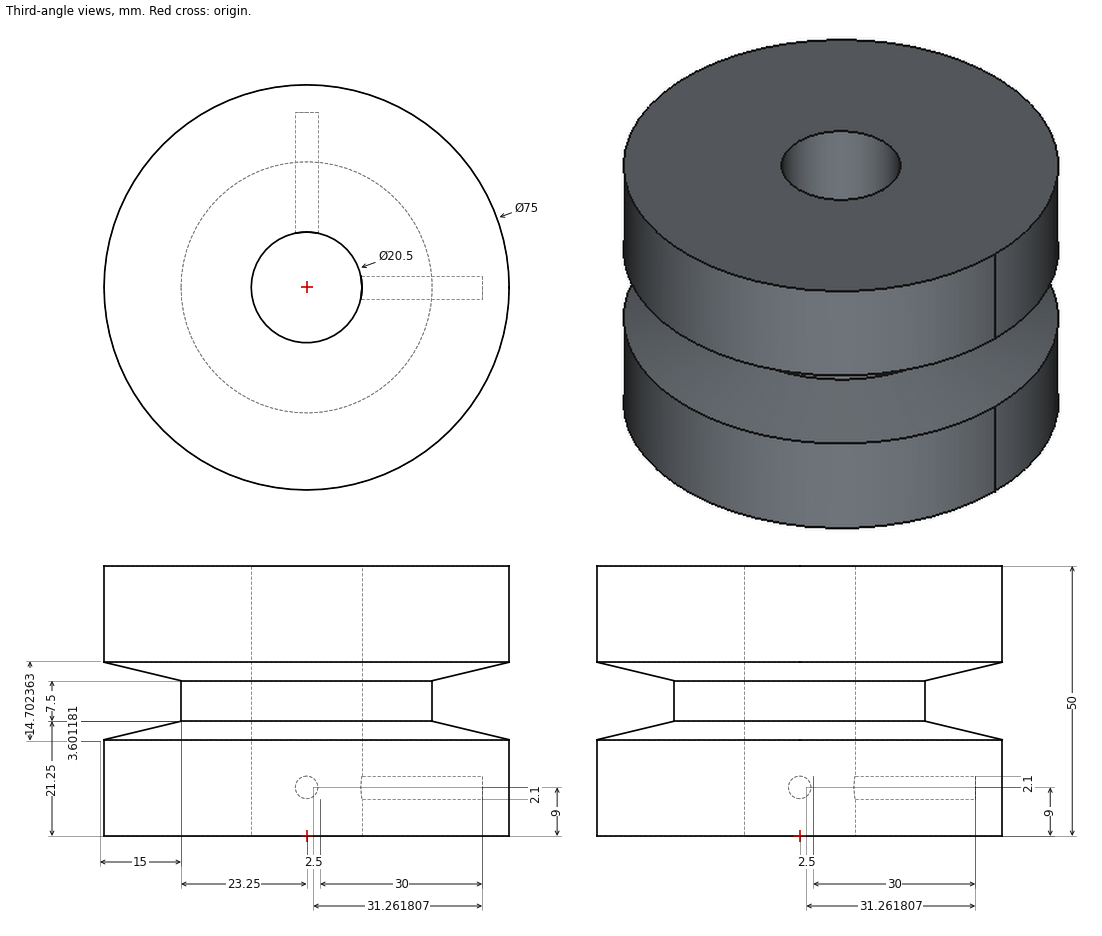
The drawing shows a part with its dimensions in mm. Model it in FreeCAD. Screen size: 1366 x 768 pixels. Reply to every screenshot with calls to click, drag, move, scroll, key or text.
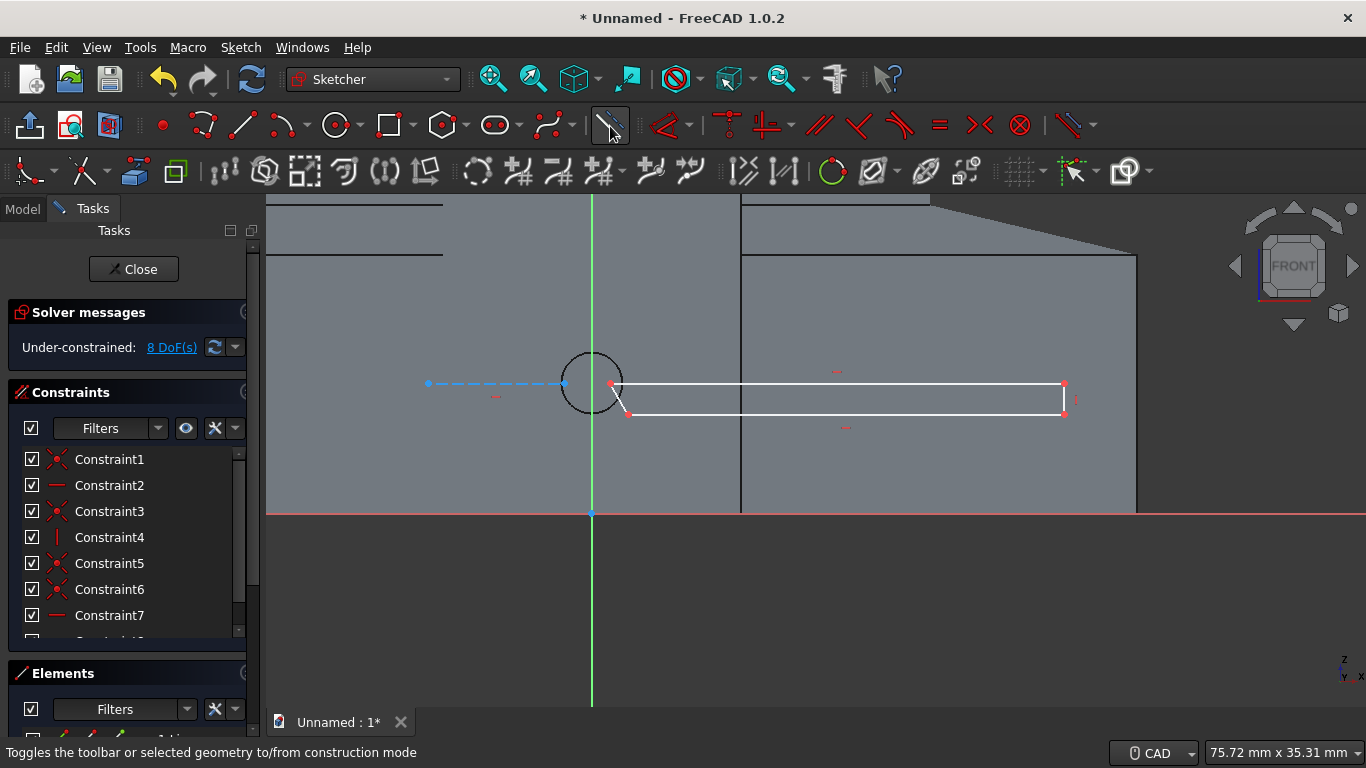
click(933, 415)
click(846, 449)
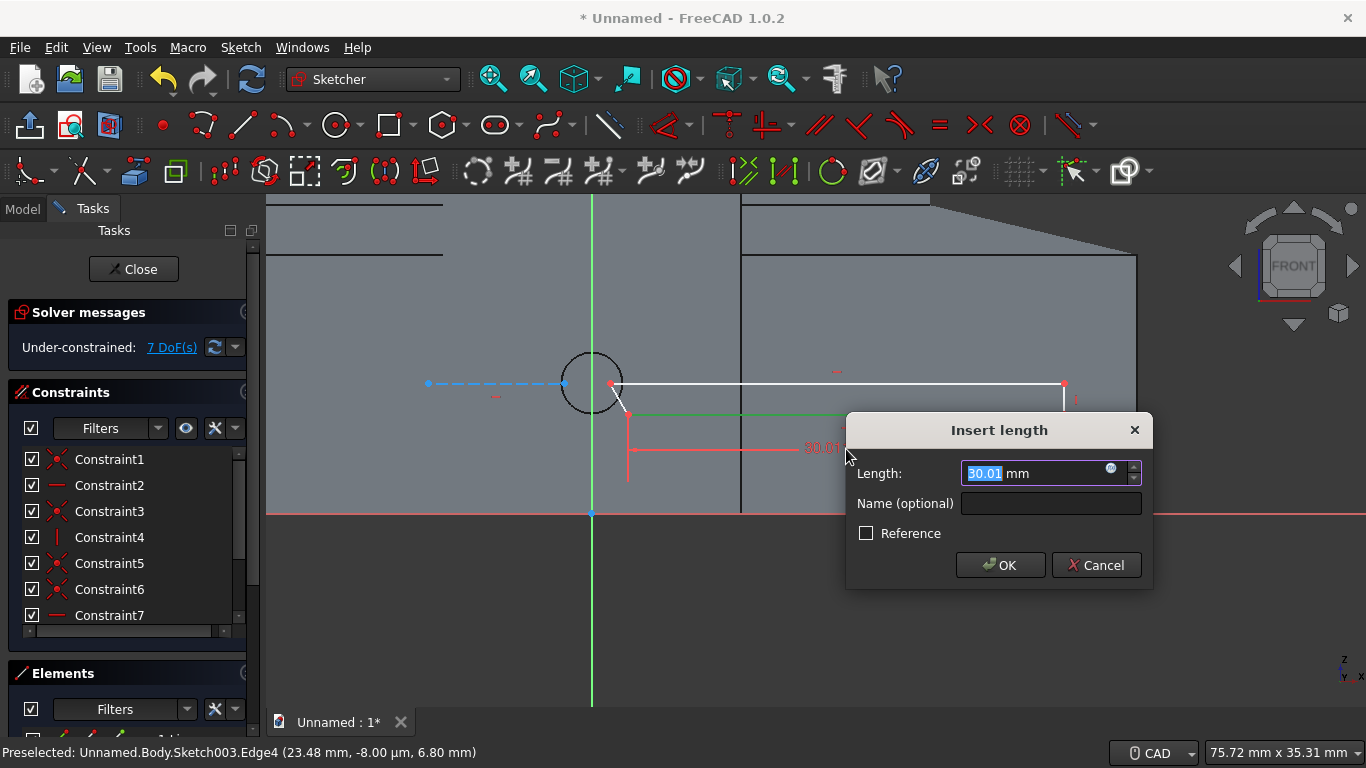
text(30)
key(Return)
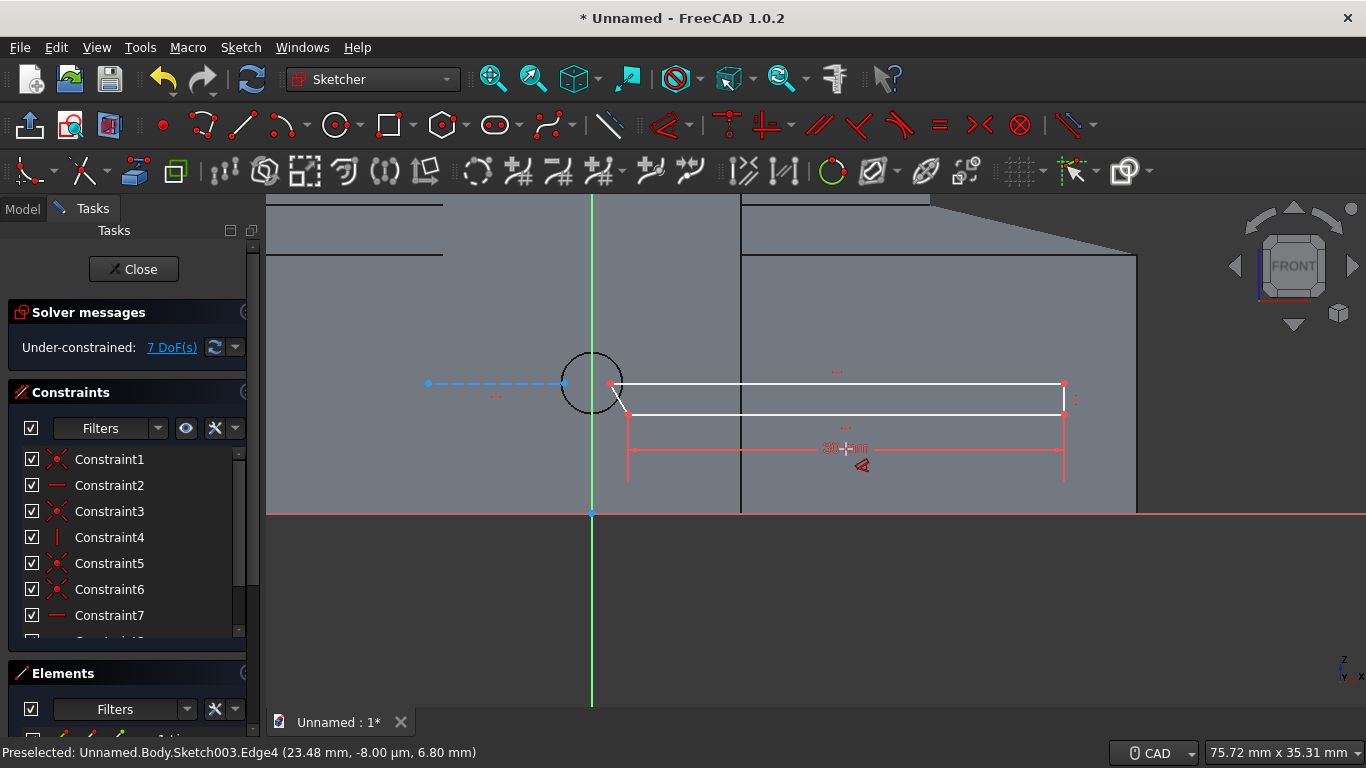
click(610, 384)
click(558, 449)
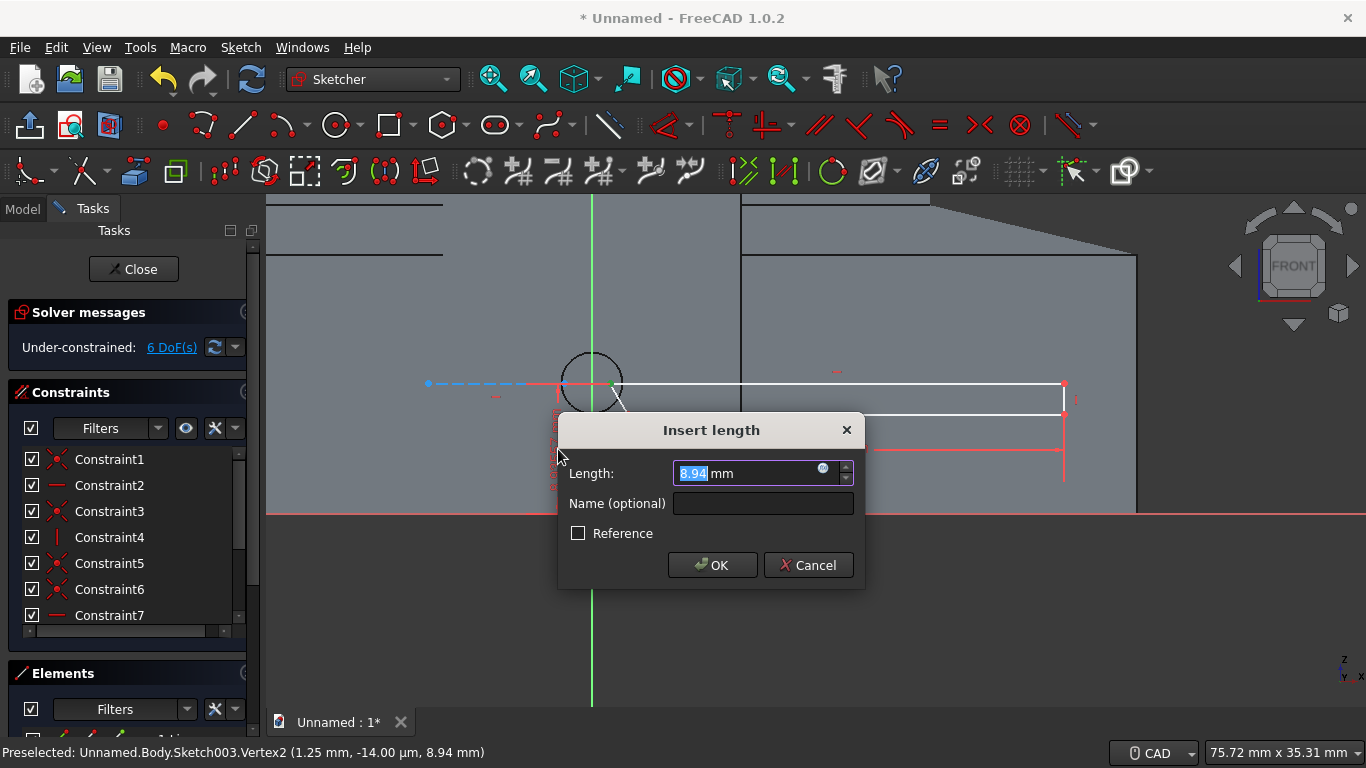
text(9)
key(Return)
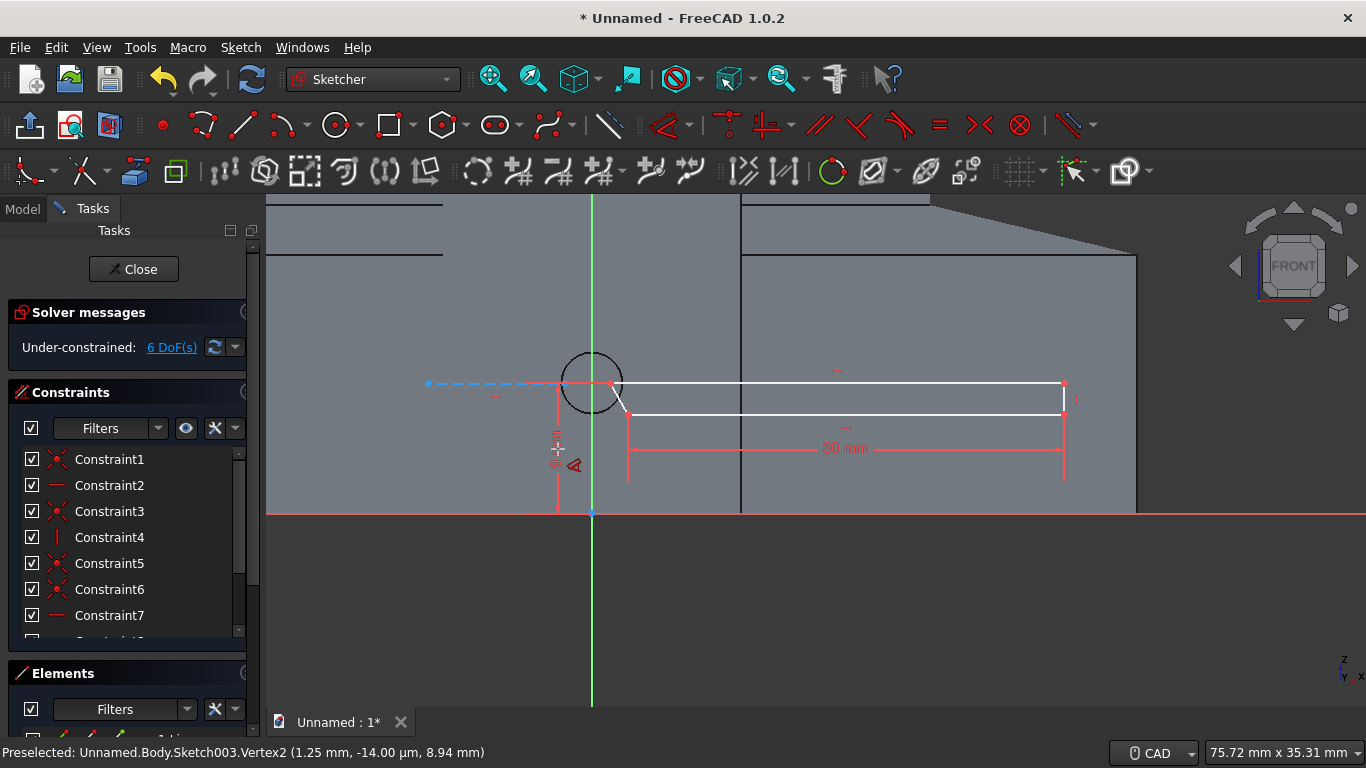
click(564, 384)
click(530, 419)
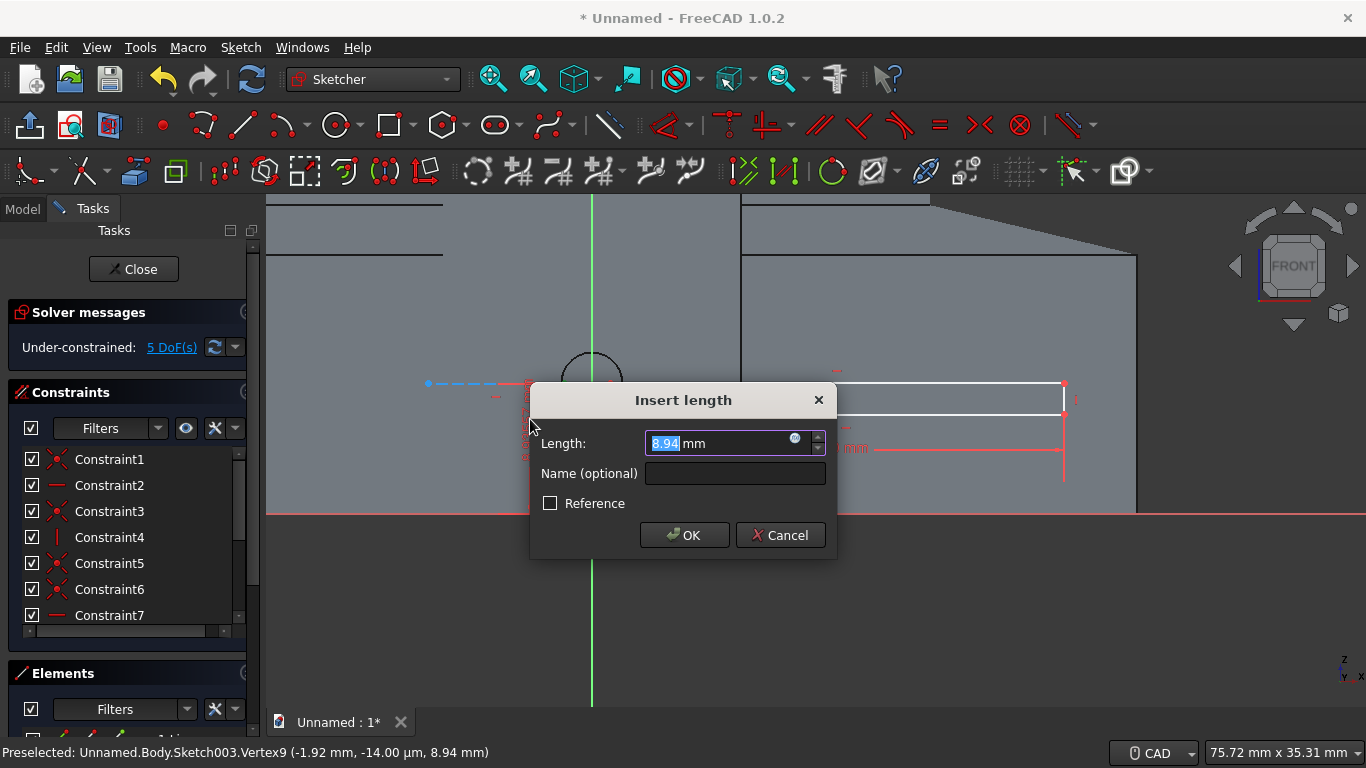
text(9)
key(Return)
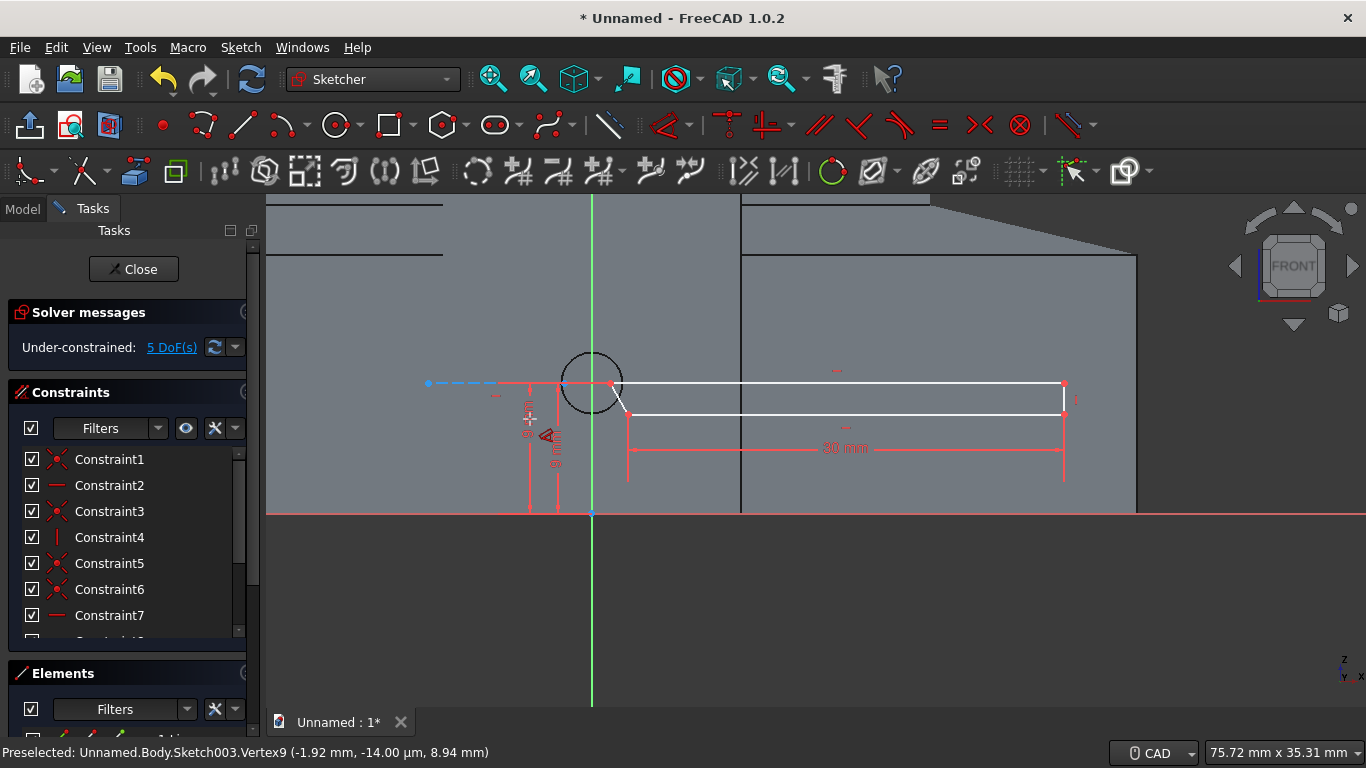
scroll(1064, 393, up, 2)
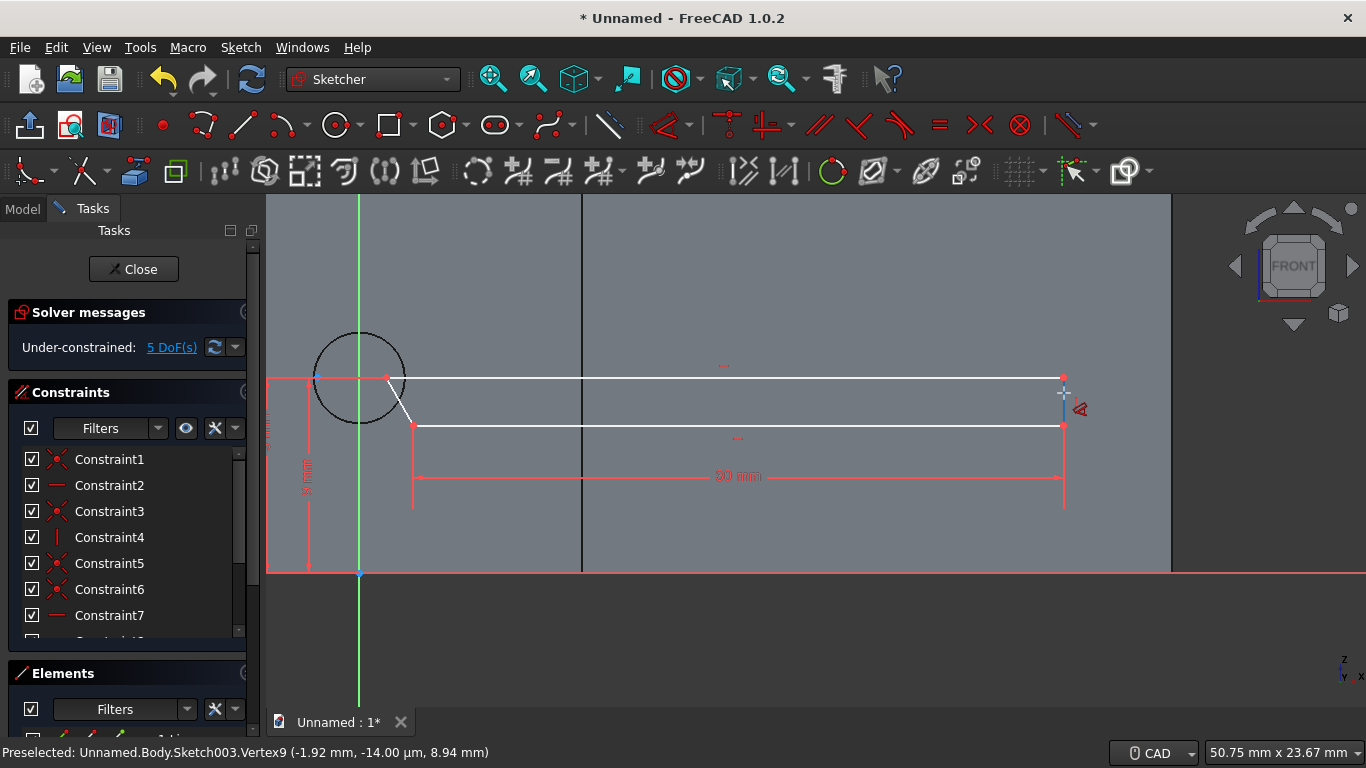
click(1064, 392)
click(1098, 402)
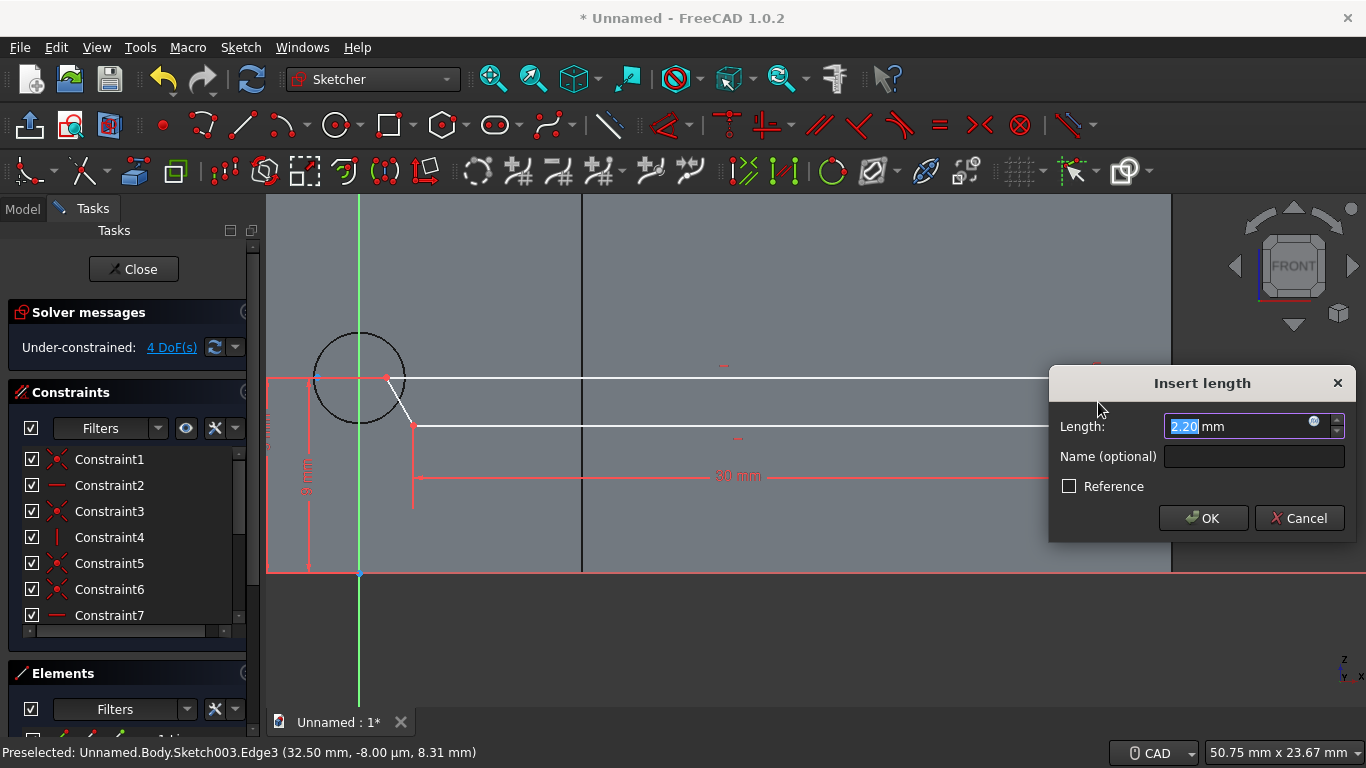
text(2.1)
key(Return)